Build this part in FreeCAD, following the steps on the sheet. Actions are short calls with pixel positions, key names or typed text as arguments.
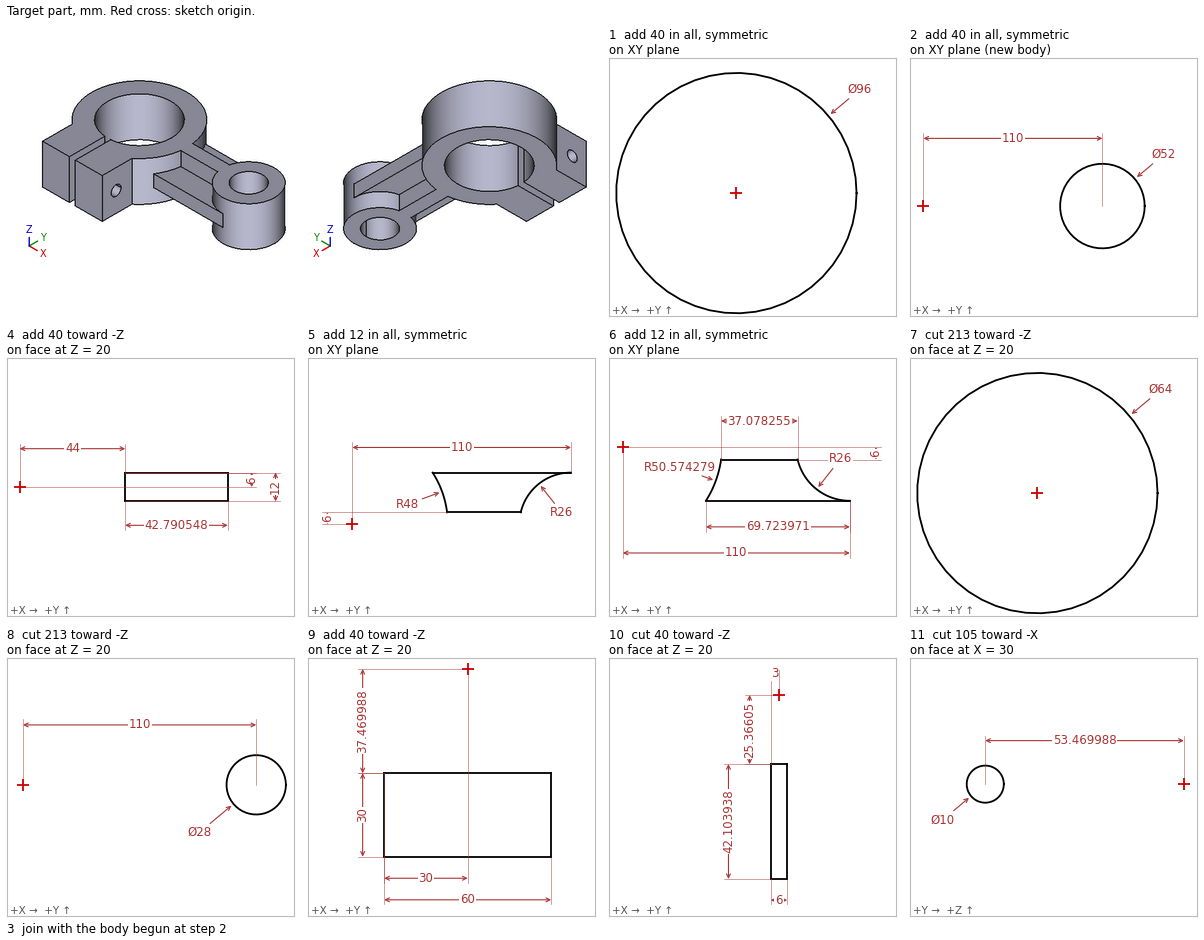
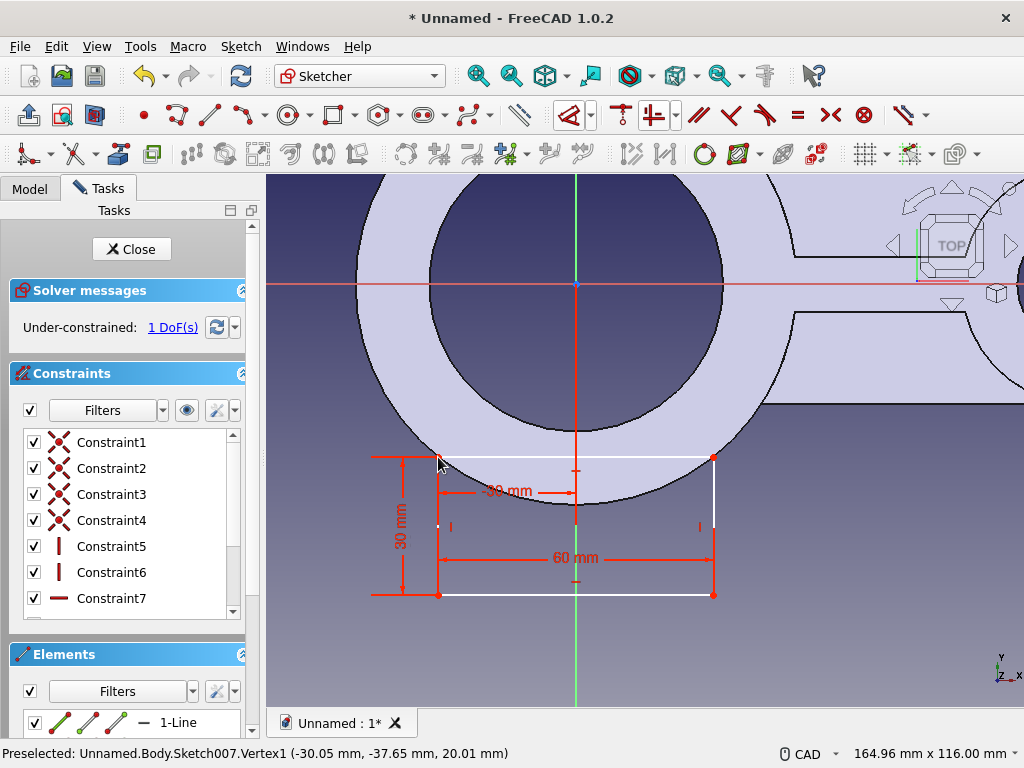
click(438, 457)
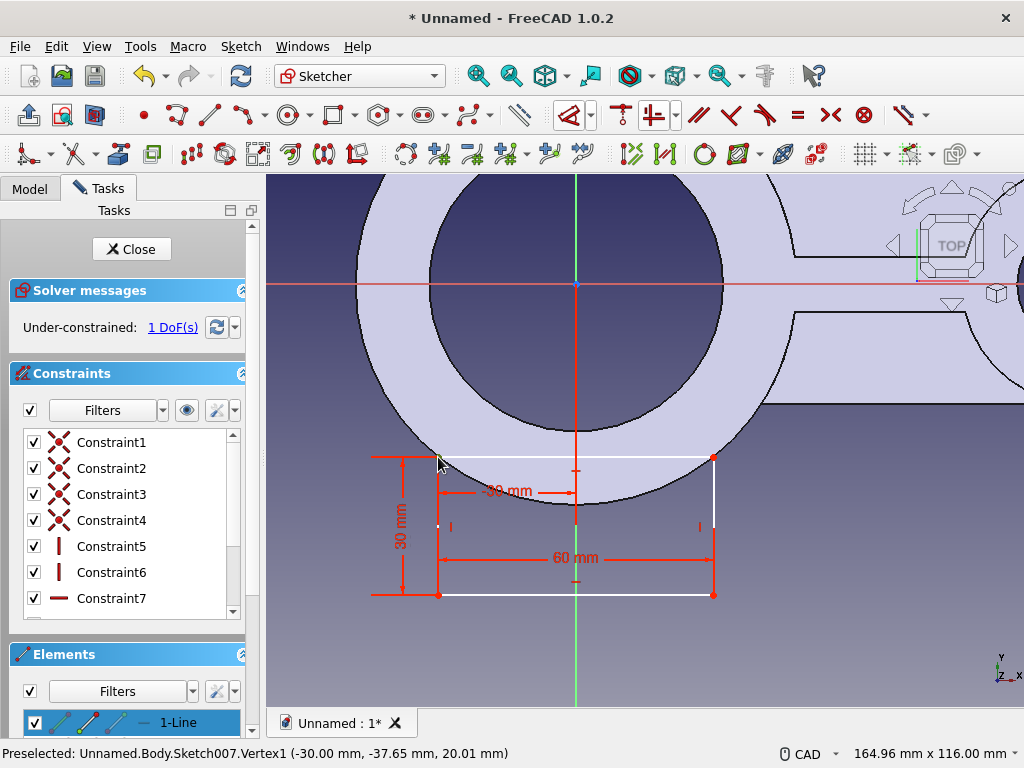
click(590, 116)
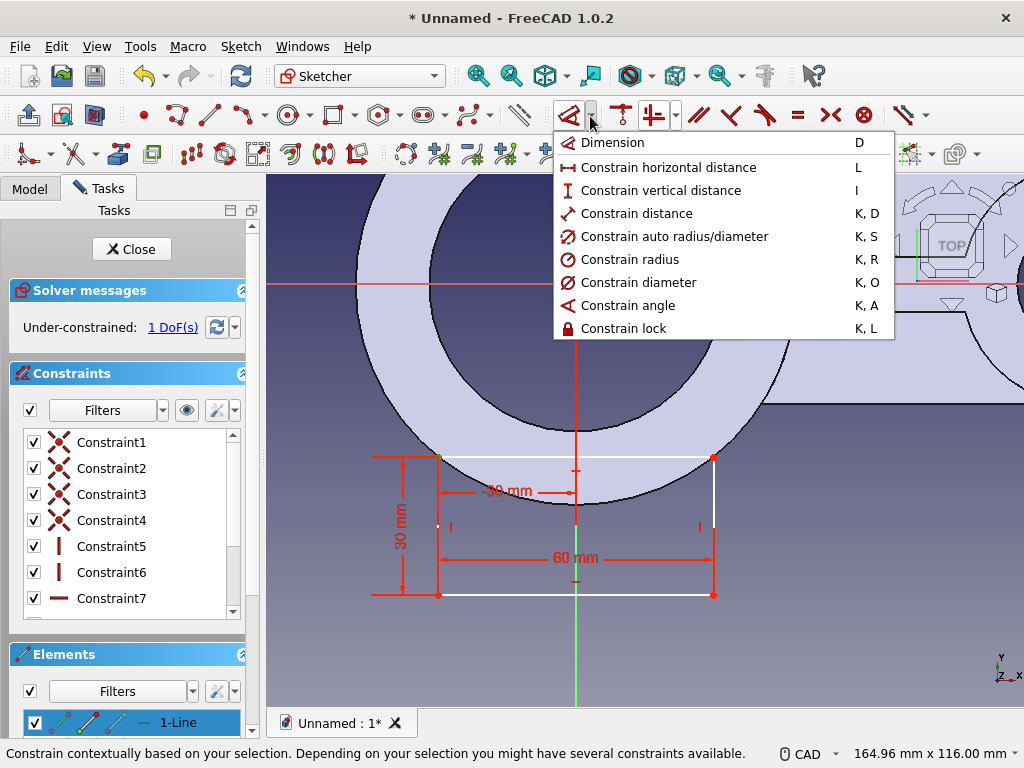
click(724, 190)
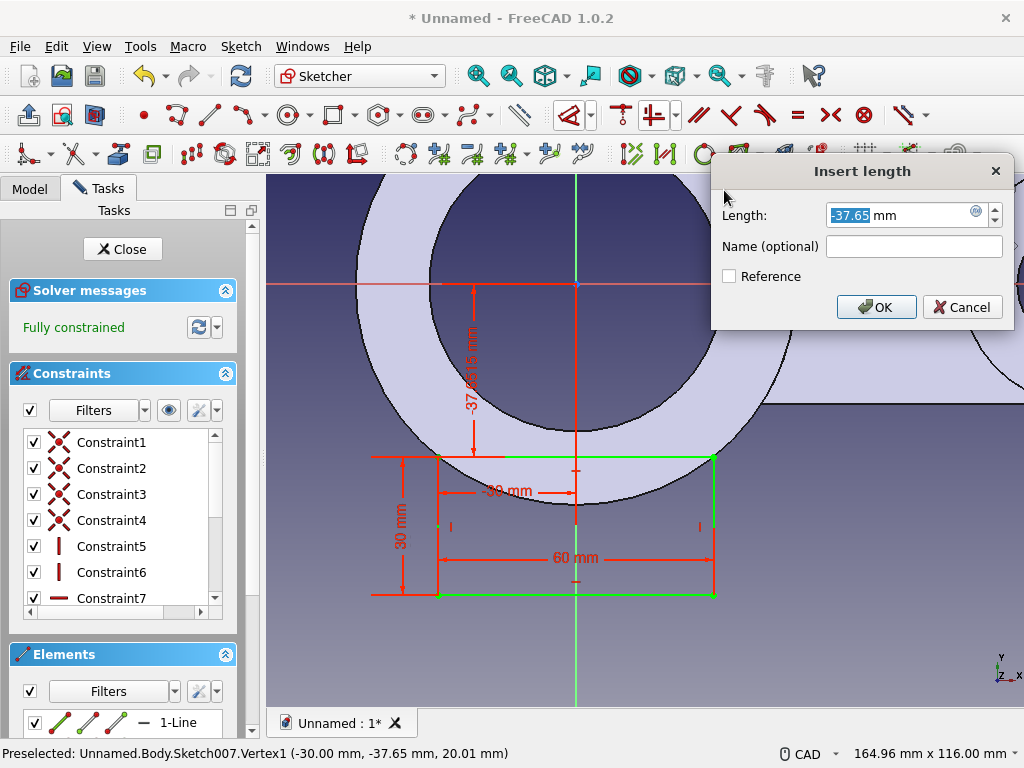
text(-37.469988)
key(Return)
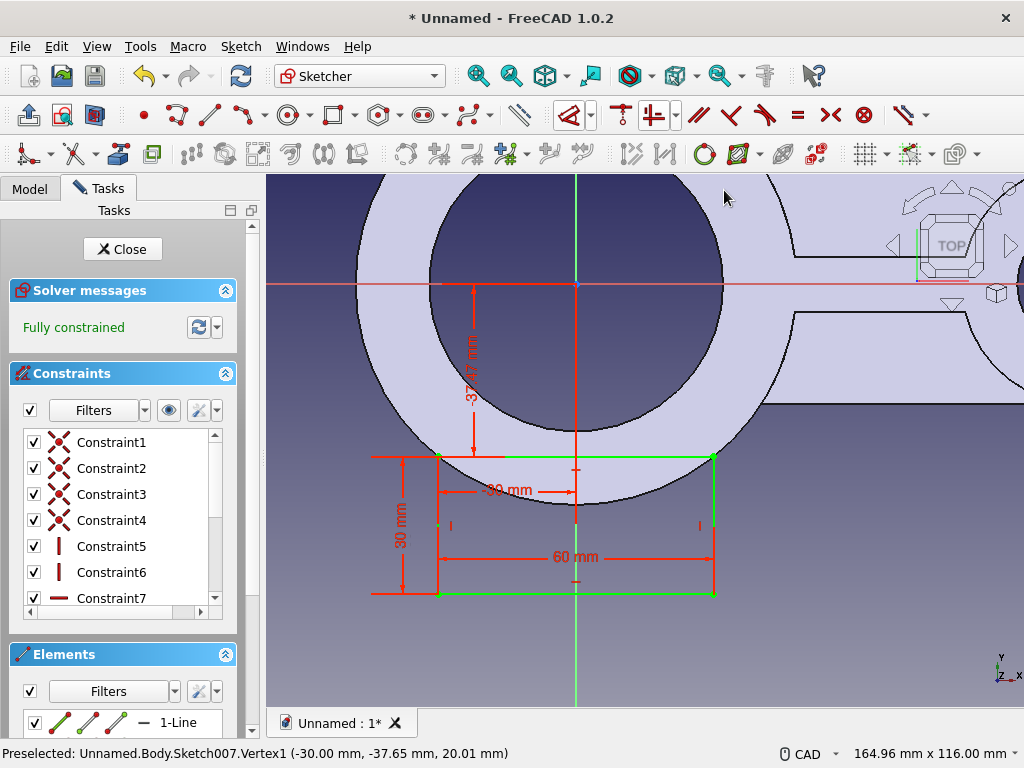
click(123, 249)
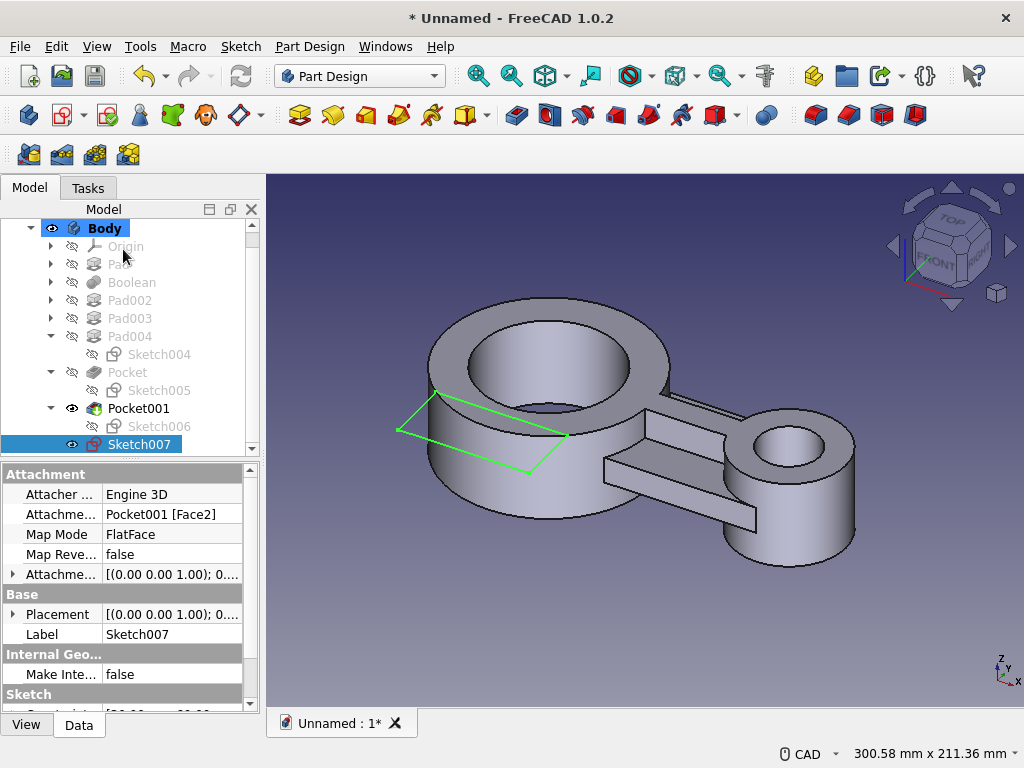
click(300, 116)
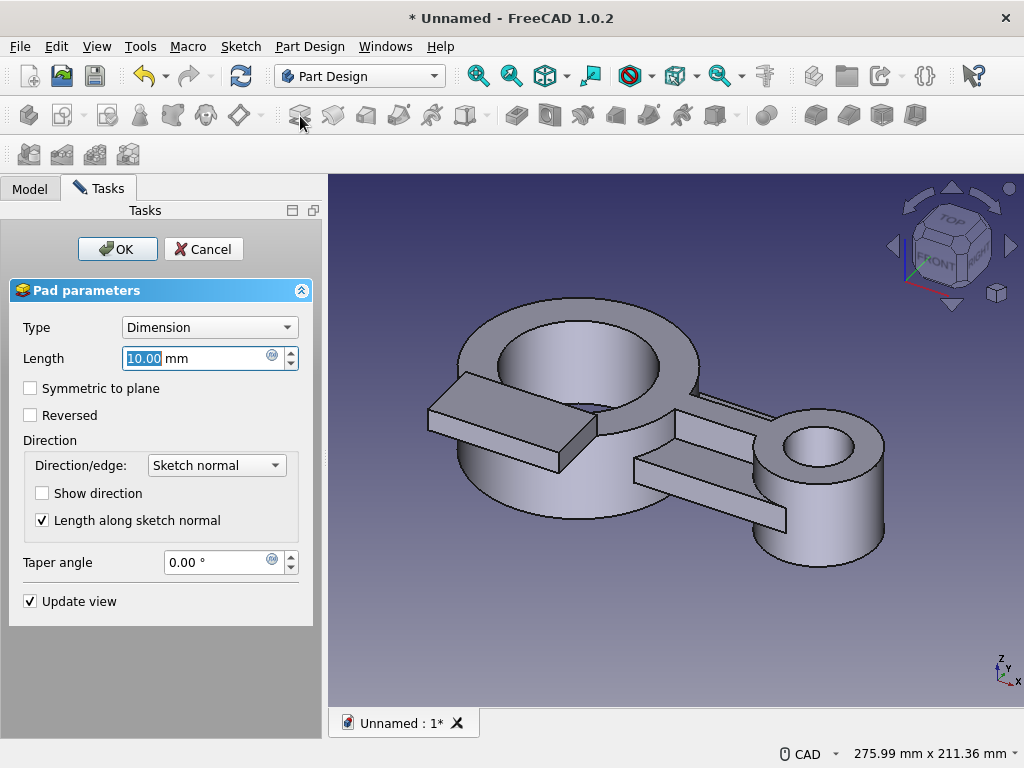
text(40)
key(Tab)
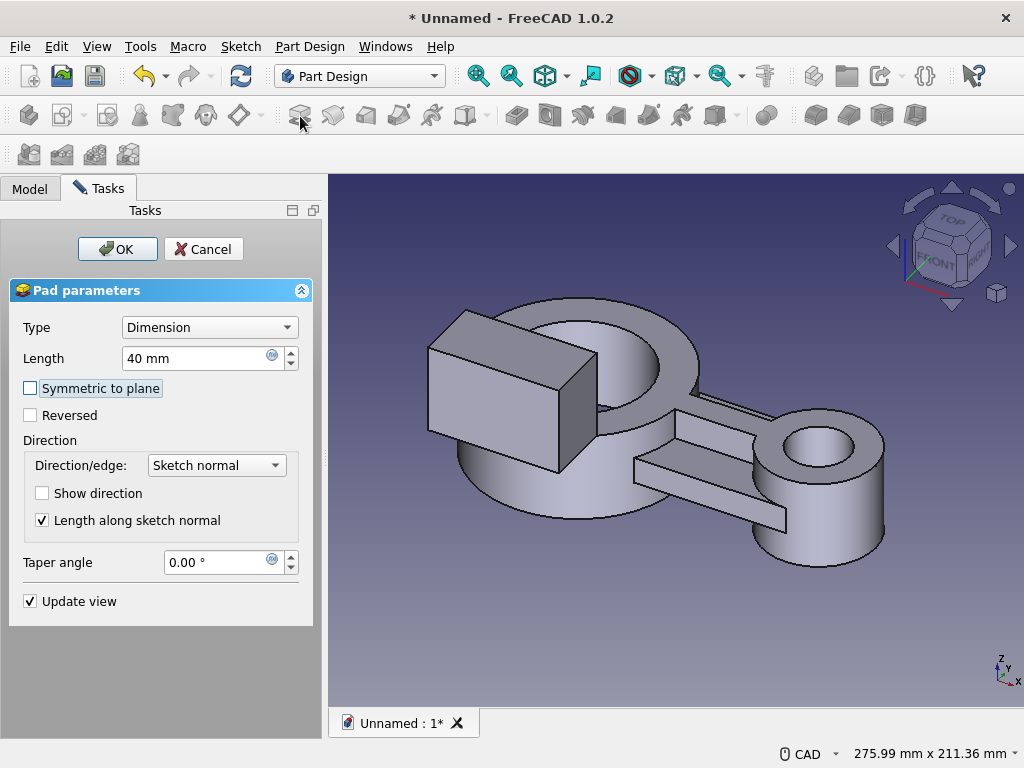
click(31, 415)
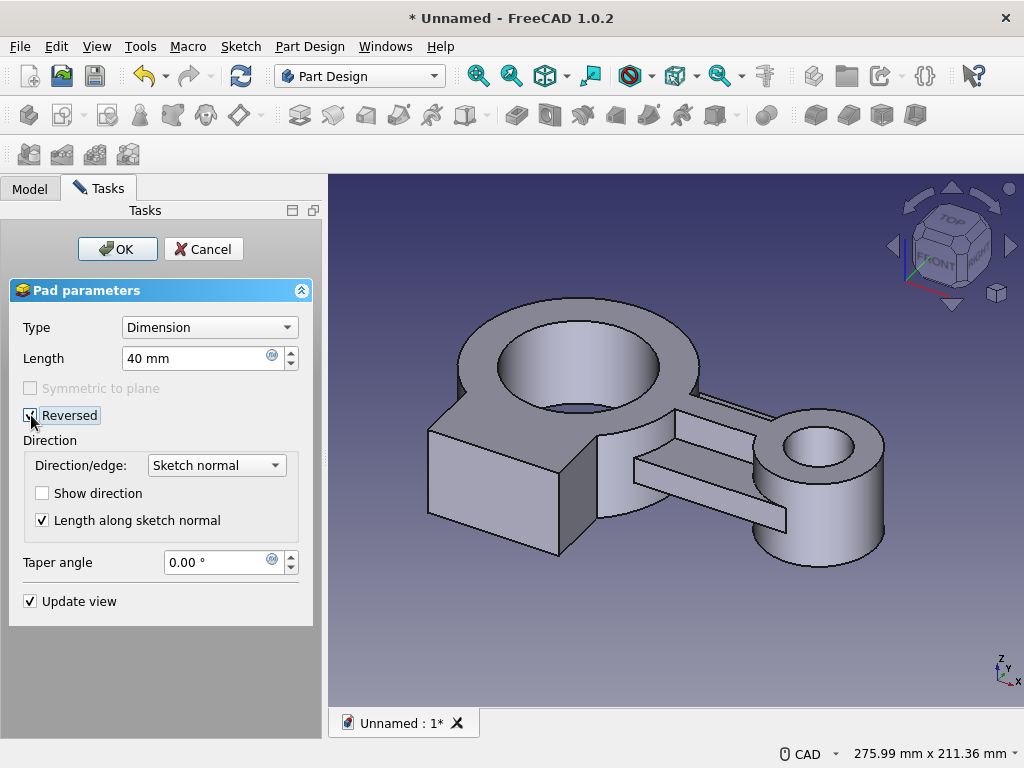
click(118, 249)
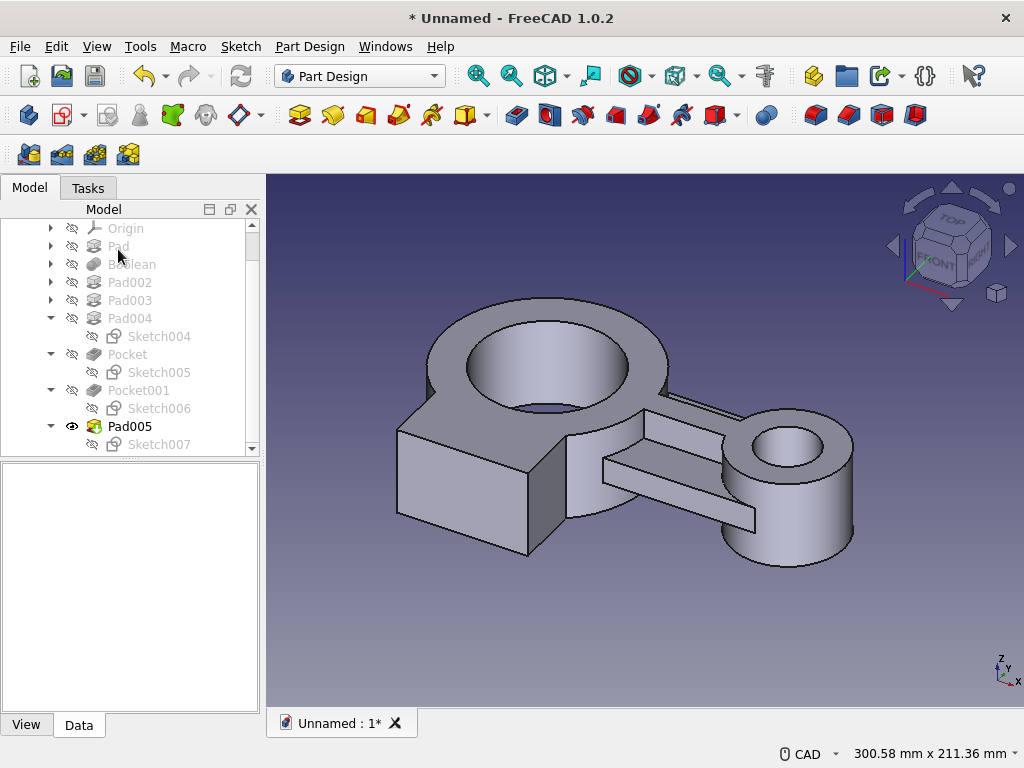
click(532, 432)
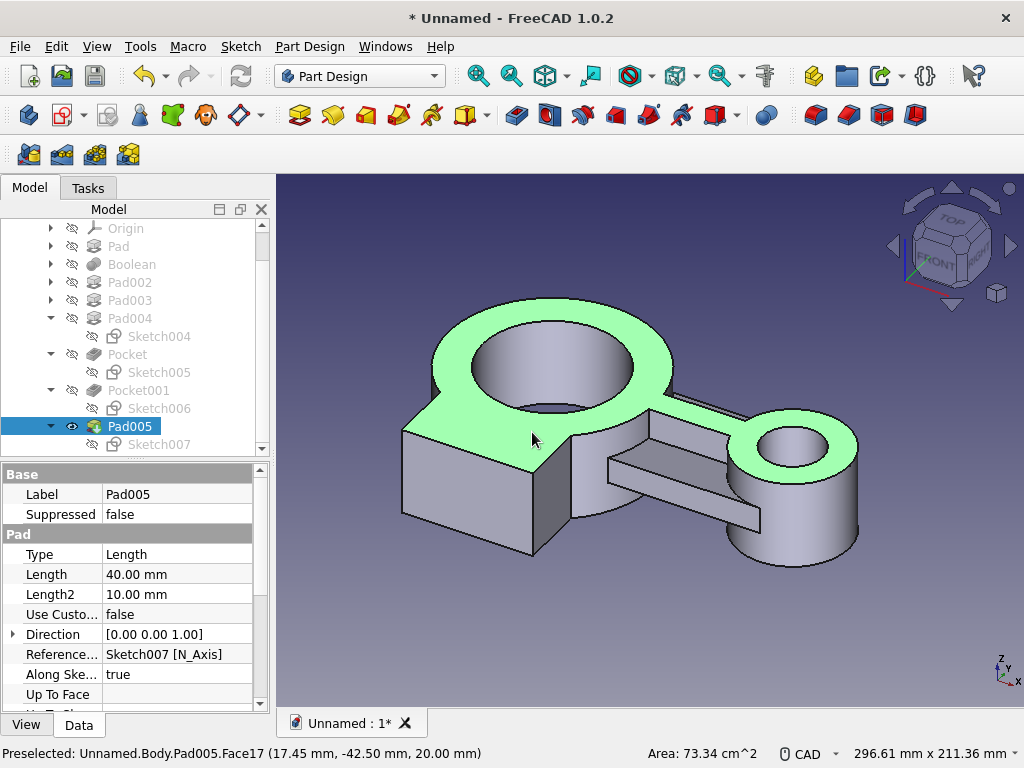
click(62, 116)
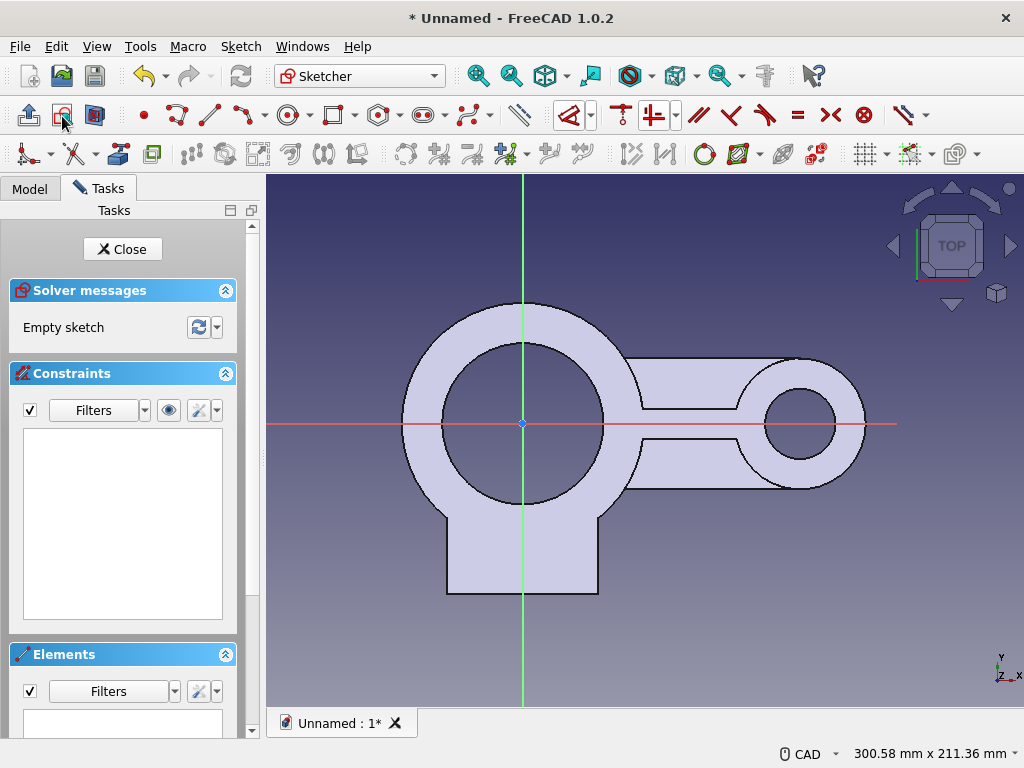
scroll(457, 592, up, 3)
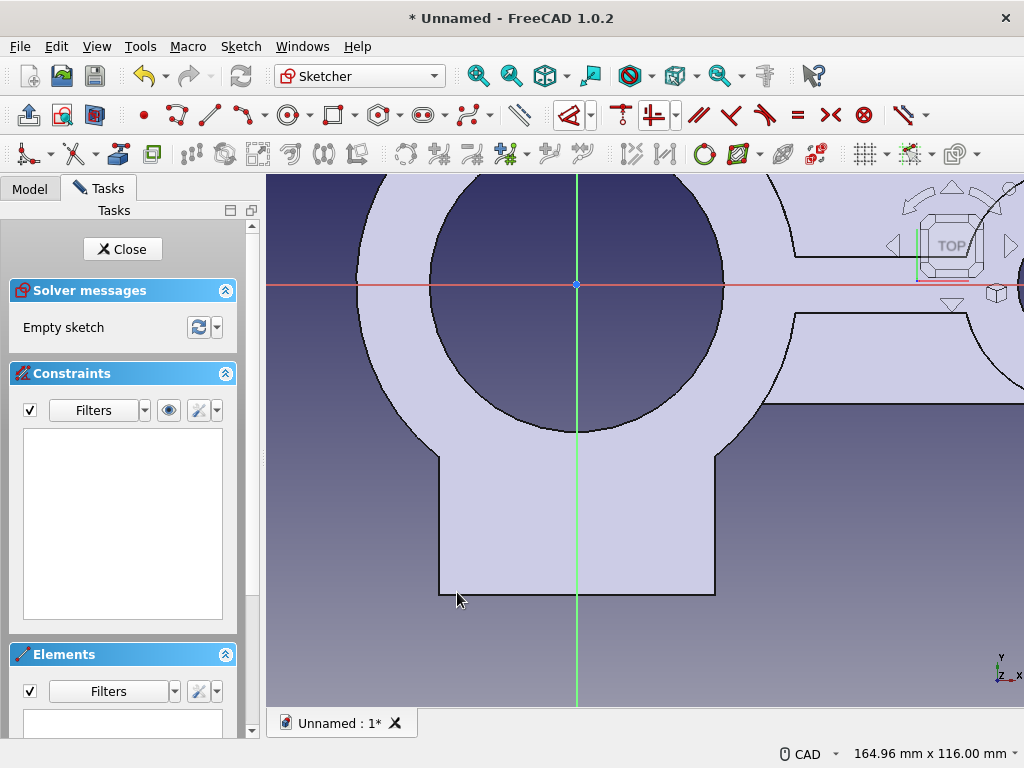
click(332, 116)